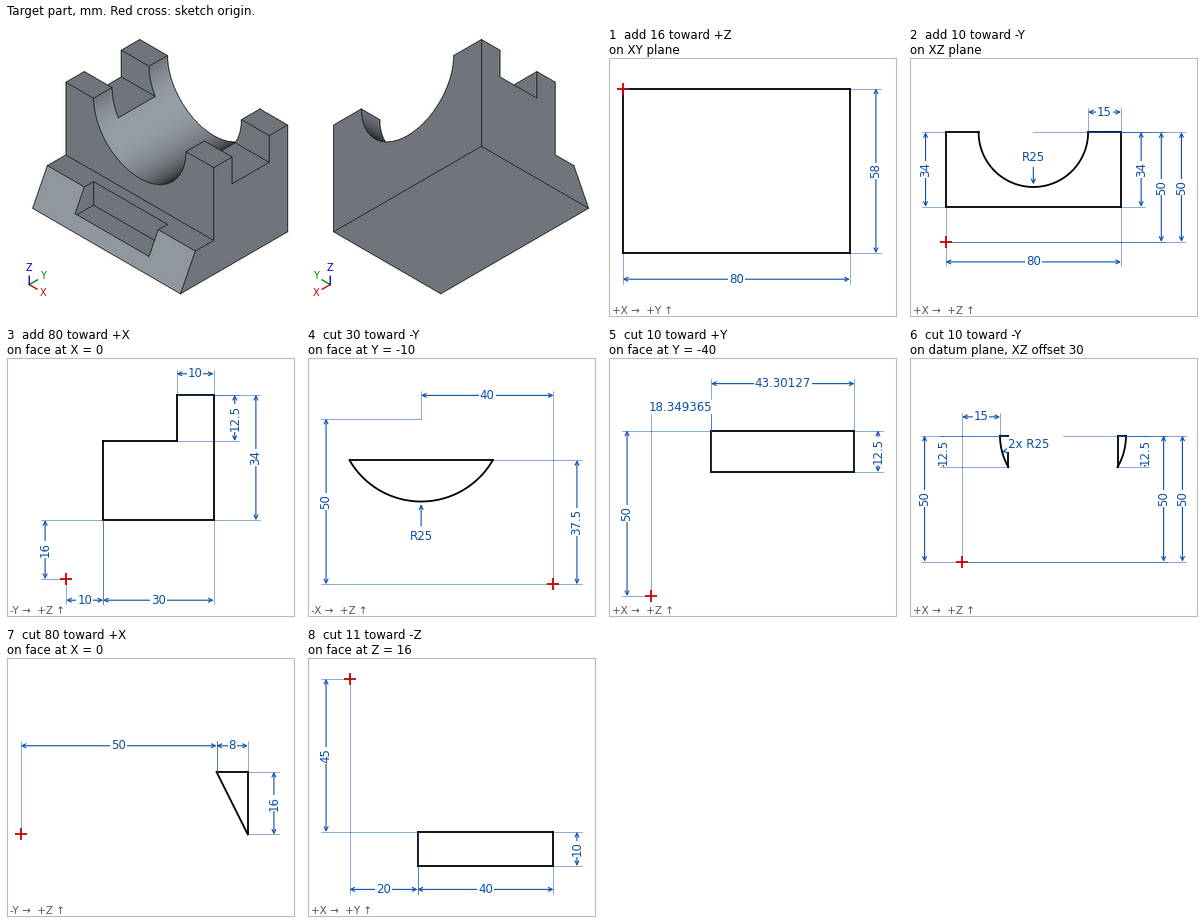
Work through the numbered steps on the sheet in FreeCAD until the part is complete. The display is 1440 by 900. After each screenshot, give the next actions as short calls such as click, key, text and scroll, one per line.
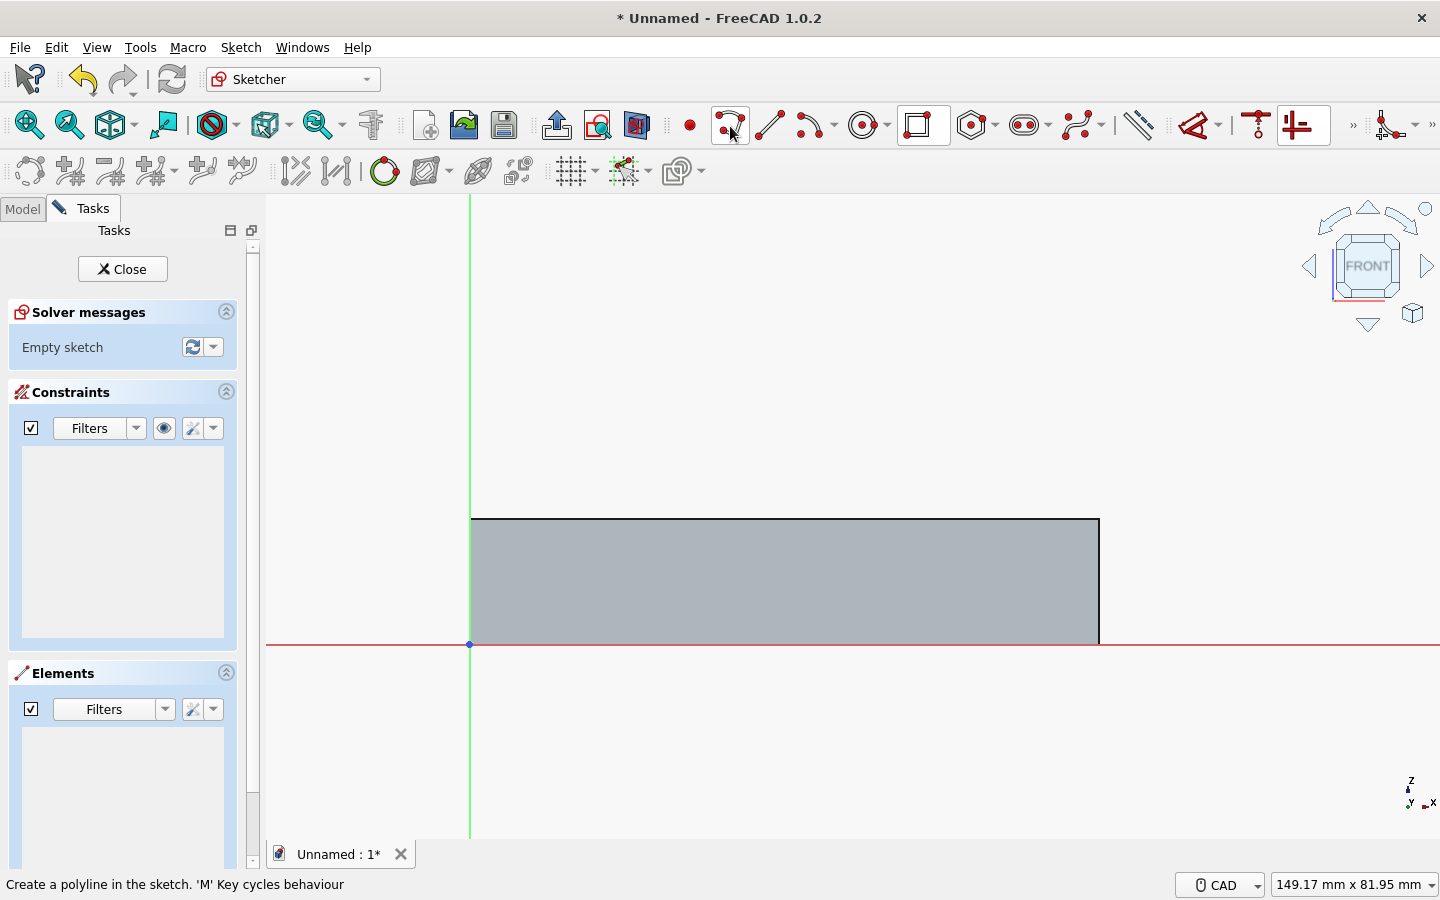
click(981, 251)
click(1099, 251)
click(1099, 519)
click(470, 519)
click(479, 251)
click(588, 251)
right_click(588, 251)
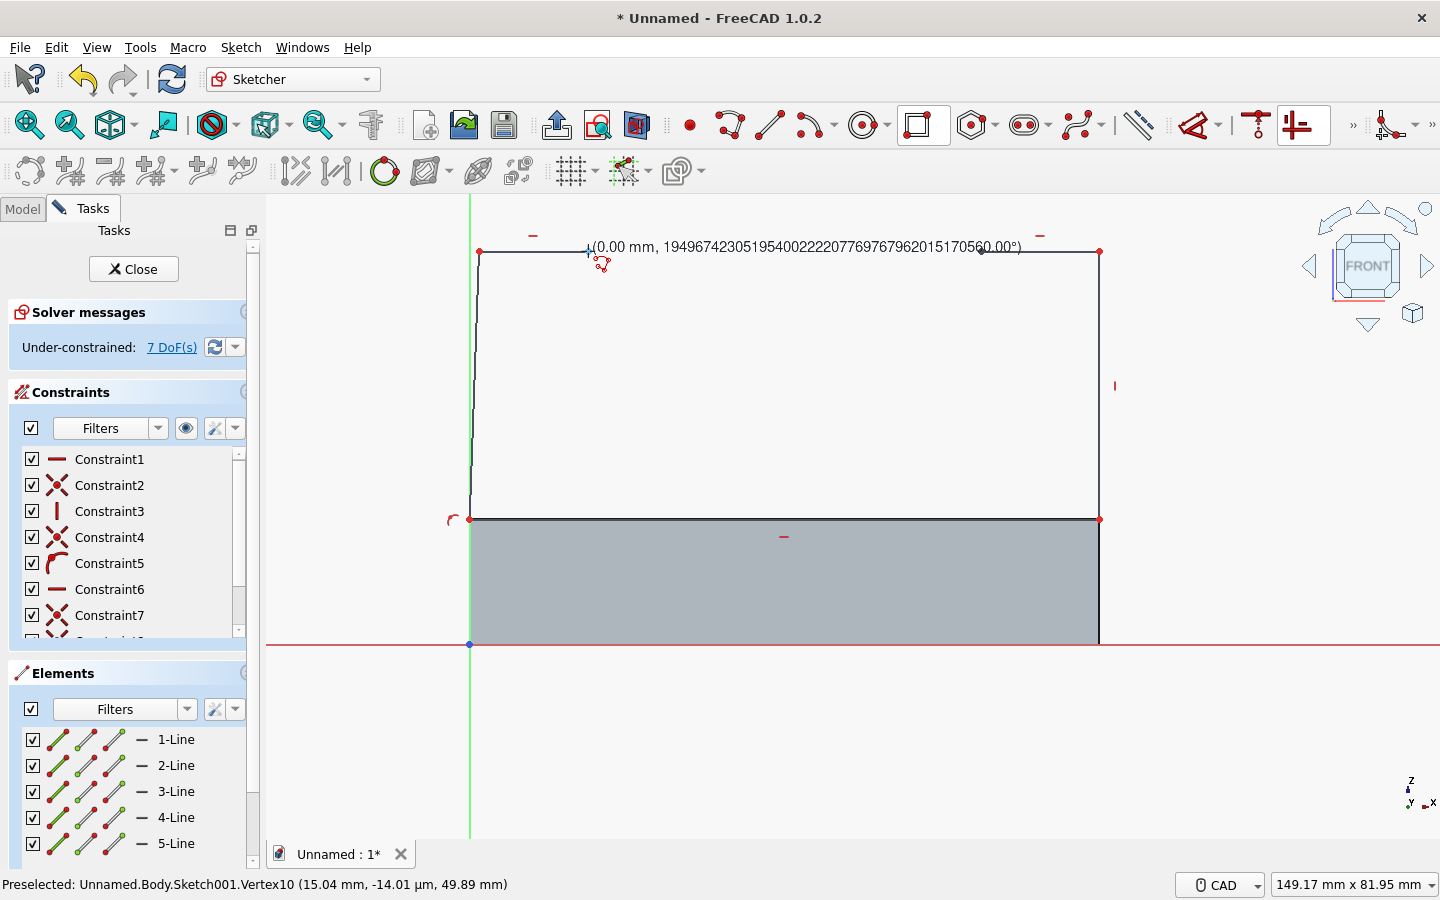
key(g)
key(3)
key(a)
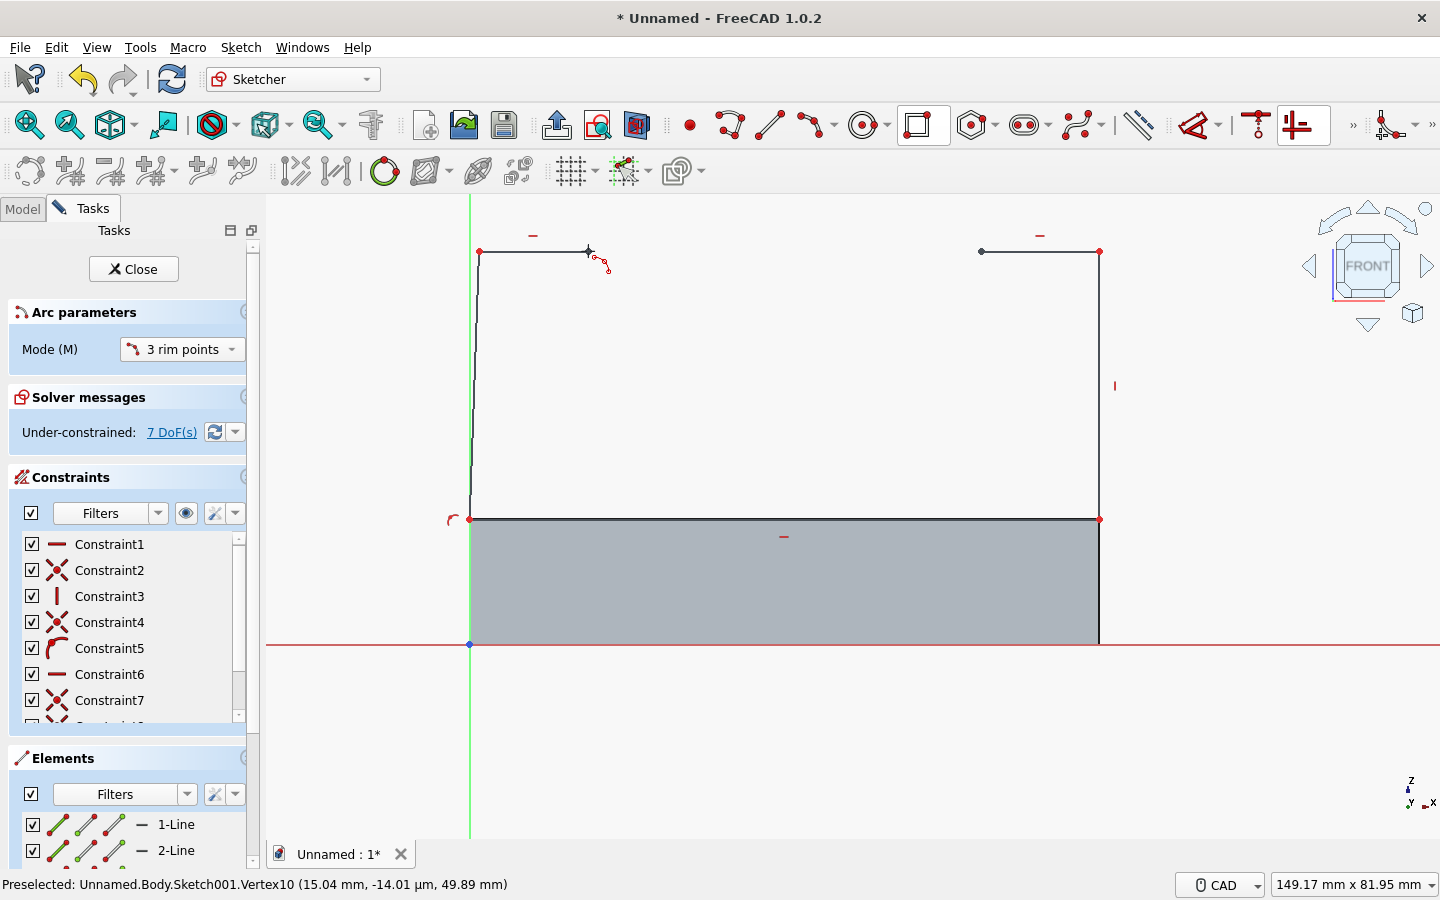
click(588, 252)
click(981, 252)
click(784, 448)
key(Escape)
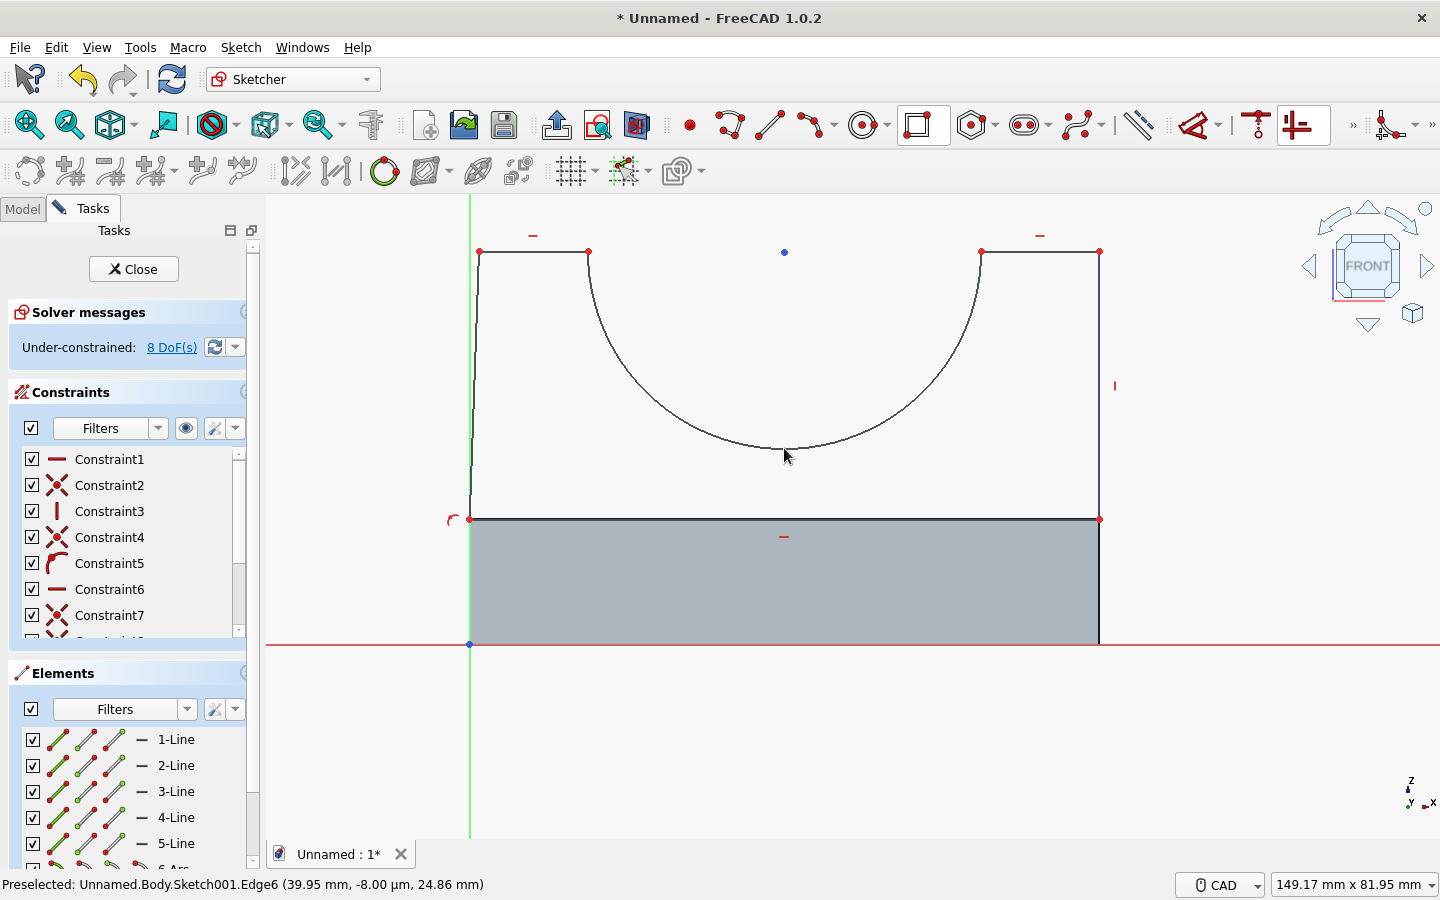
click(472, 440)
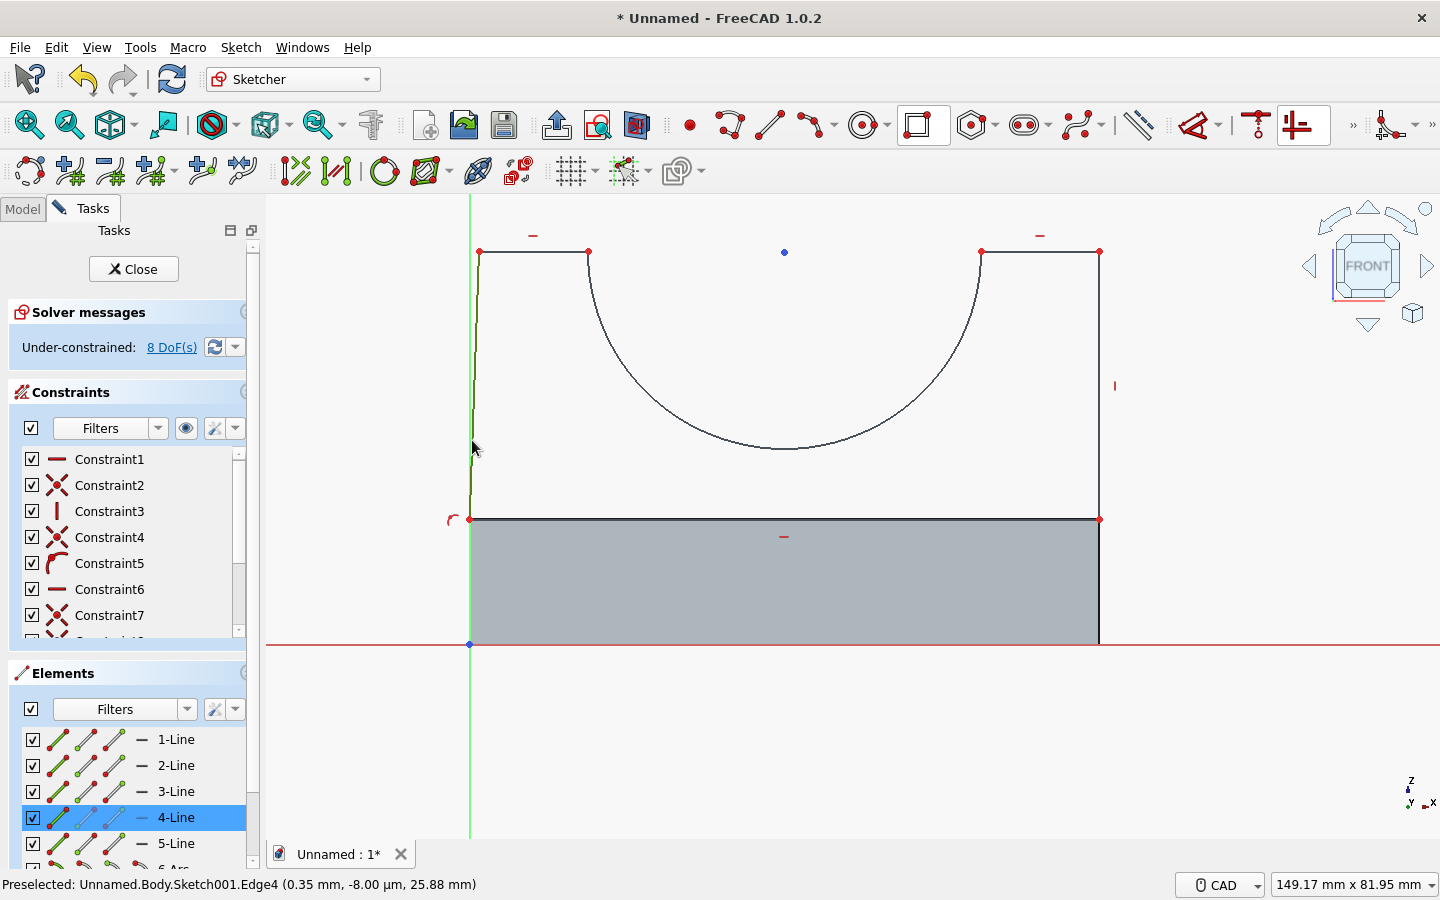
key(v)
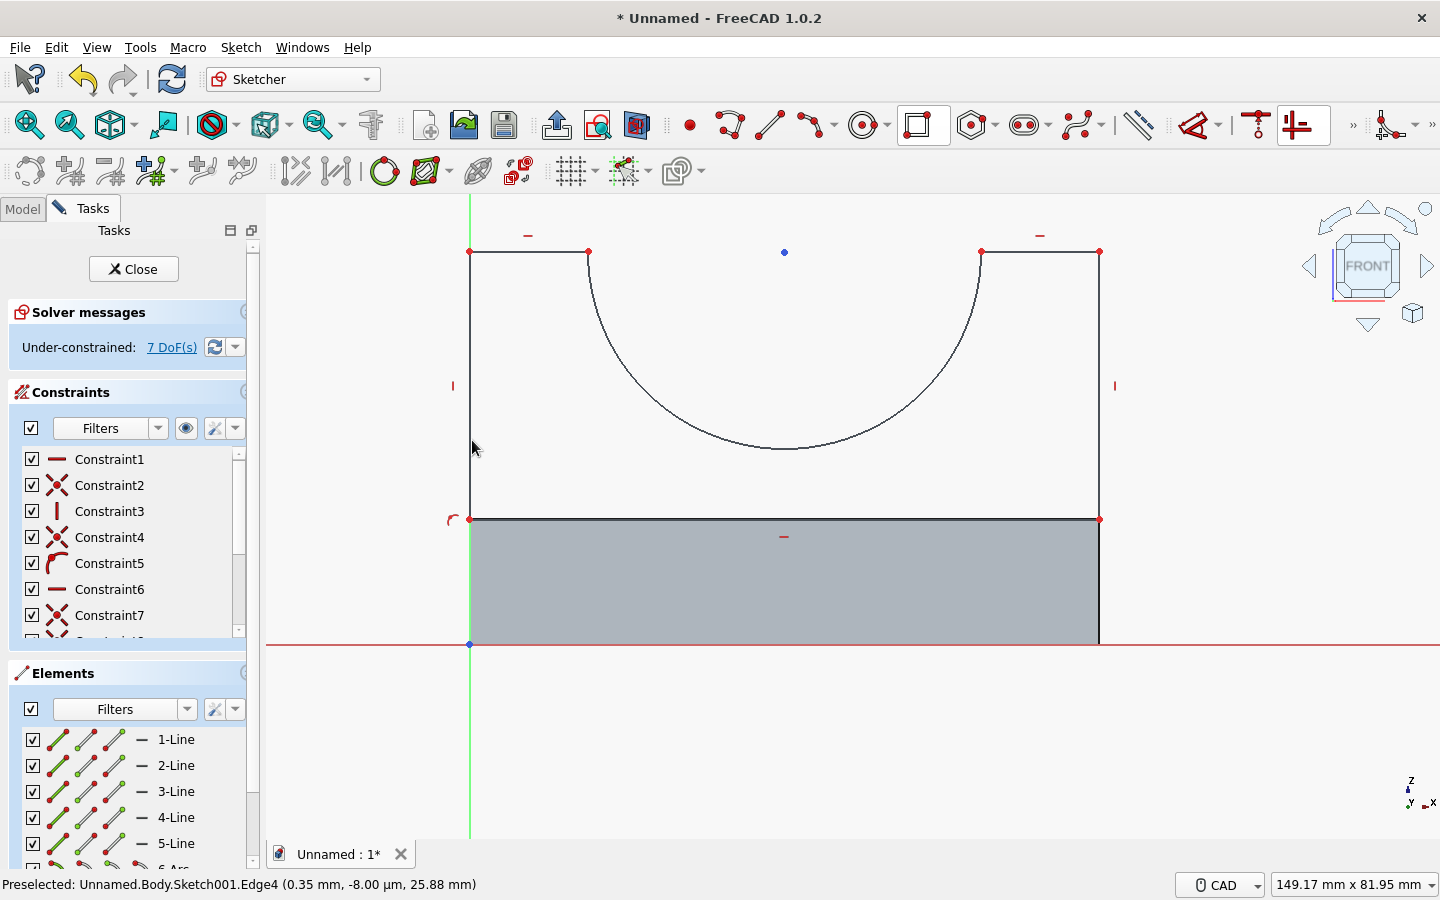
click(1194, 126)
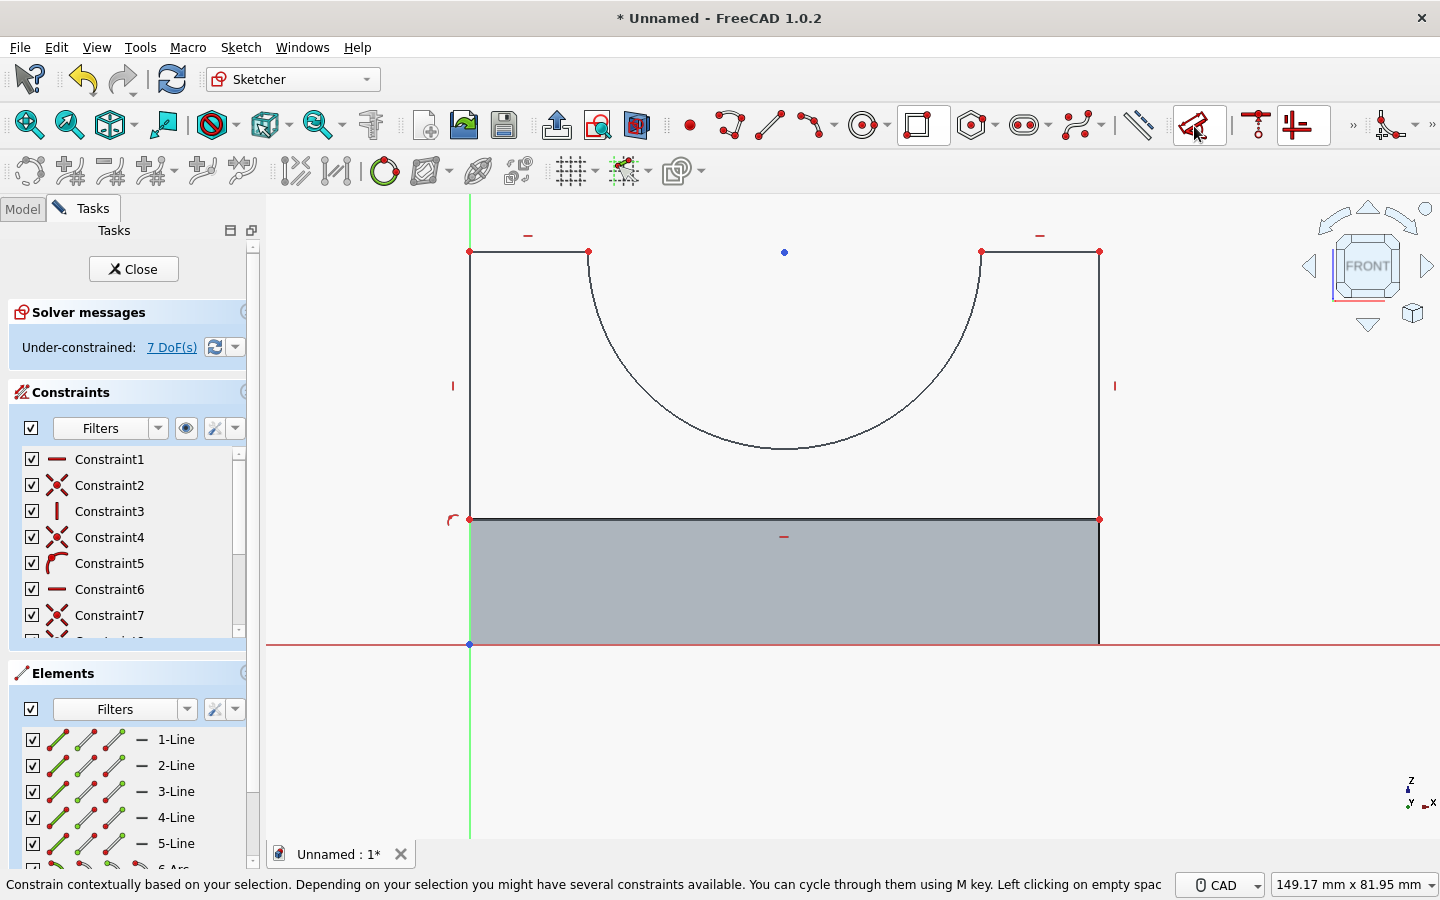
click(669, 411)
click(650, 437)